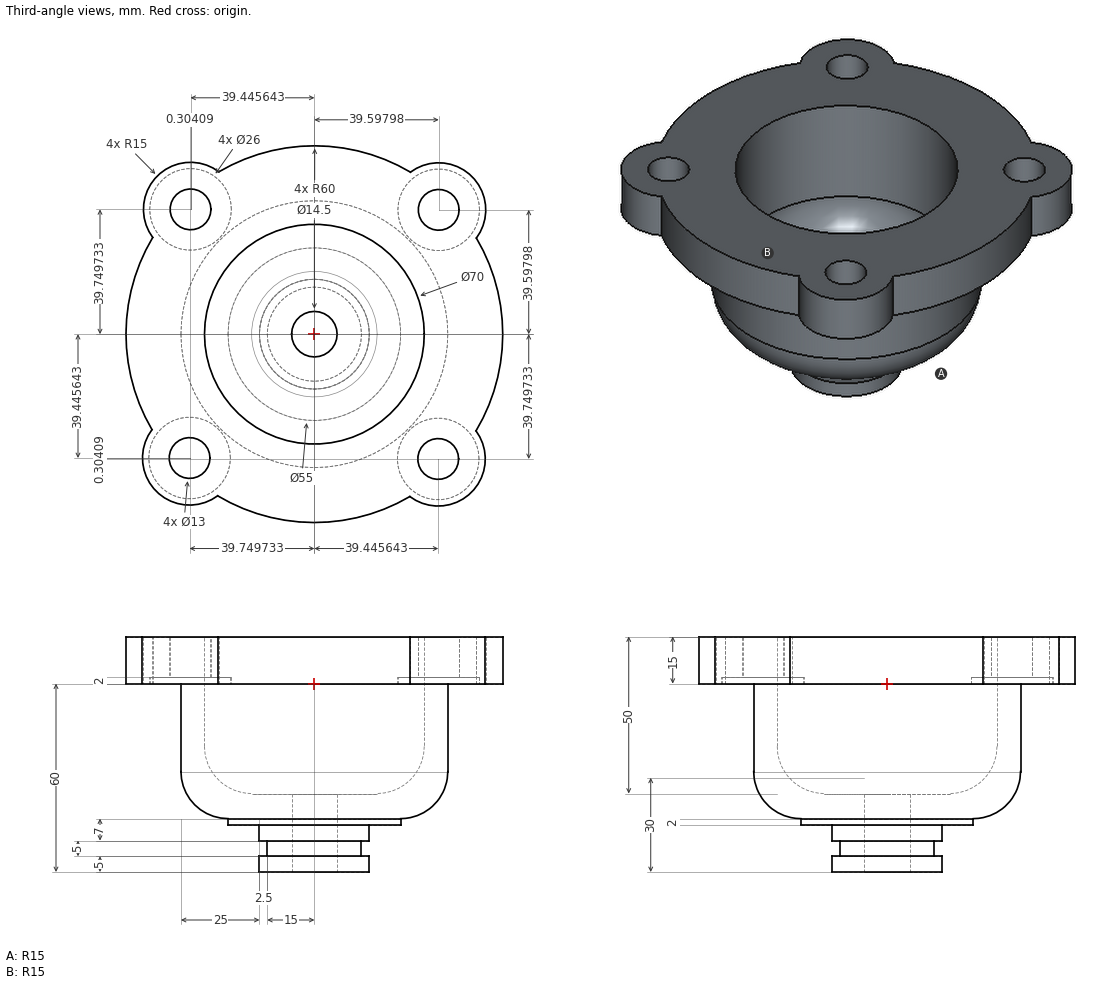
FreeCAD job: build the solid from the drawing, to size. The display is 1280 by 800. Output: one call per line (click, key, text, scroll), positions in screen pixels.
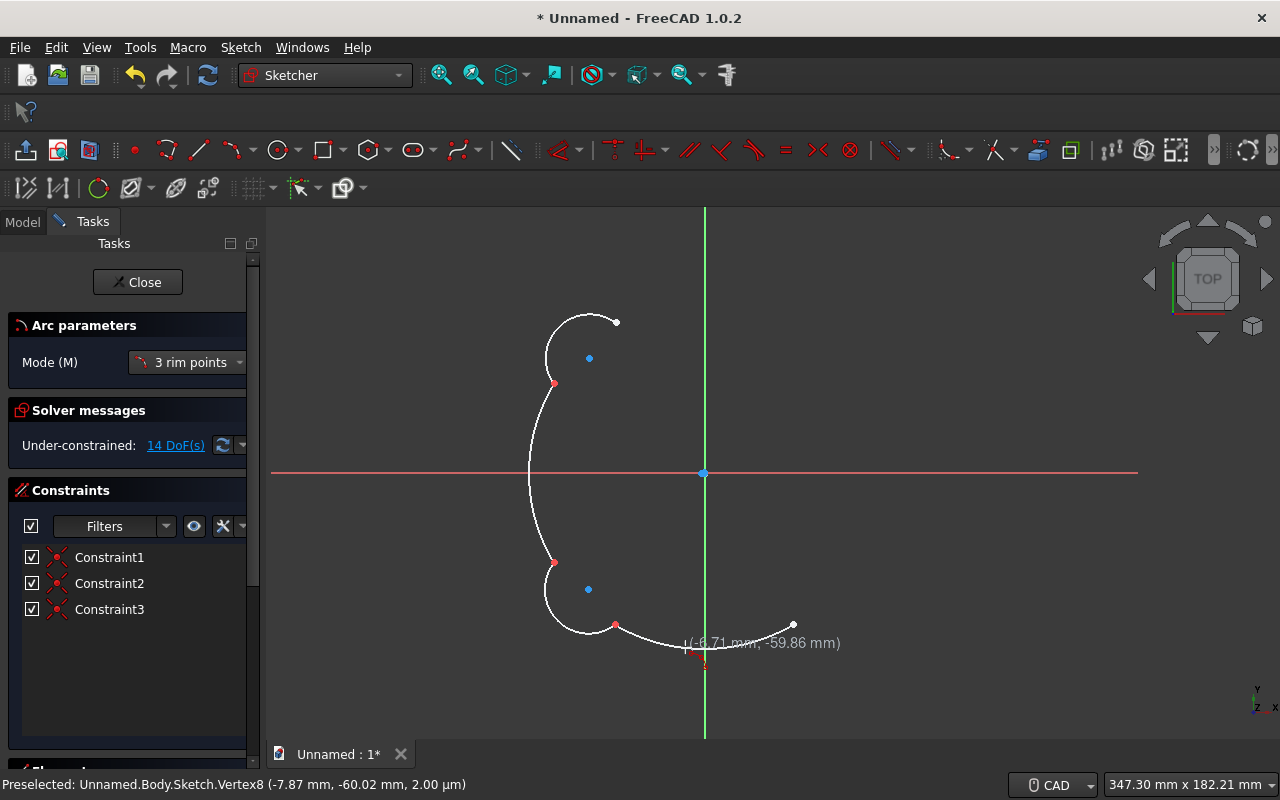
click(793, 625)
click(855, 563)
click(851, 620)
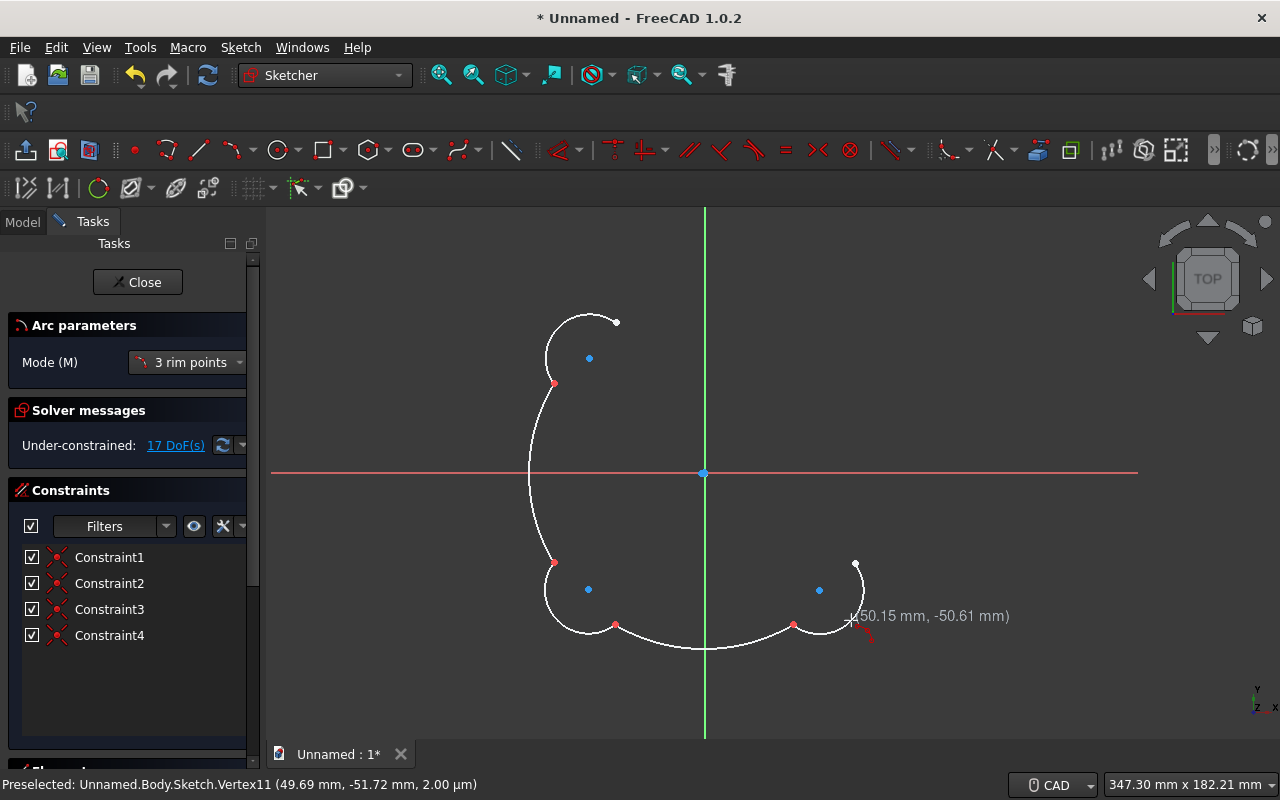
click(855, 564)
click(855, 384)
click(879, 492)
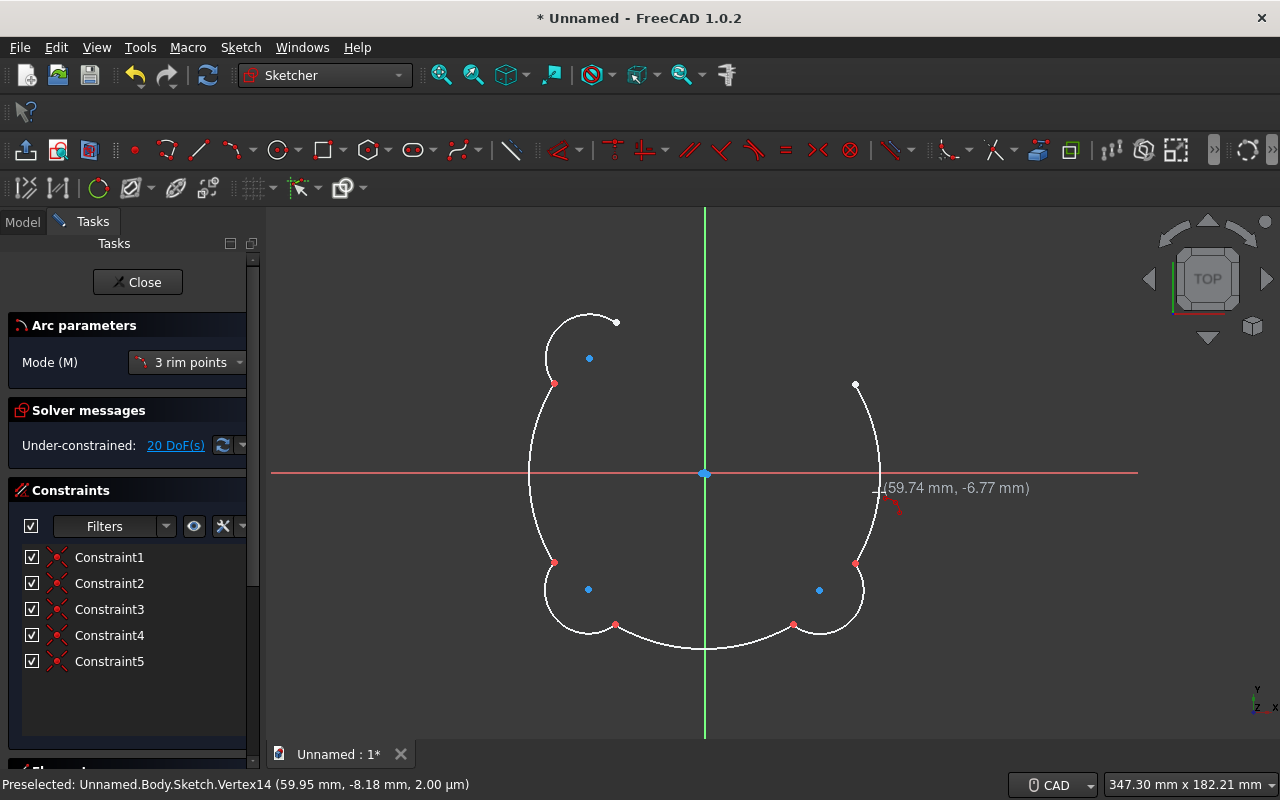
click(855, 385)
click(794, 323)
click(851, 327)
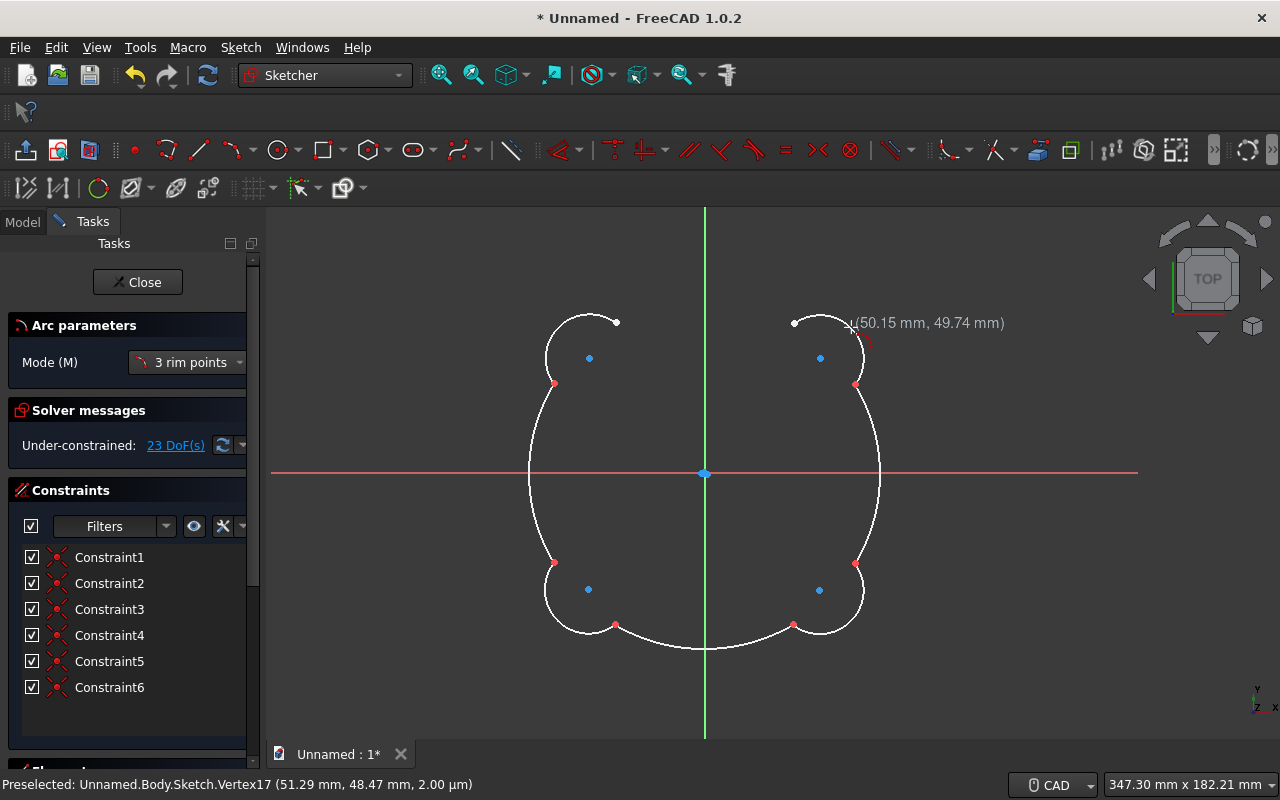
click(794, 324)
click(616, 323)
click(724, 299)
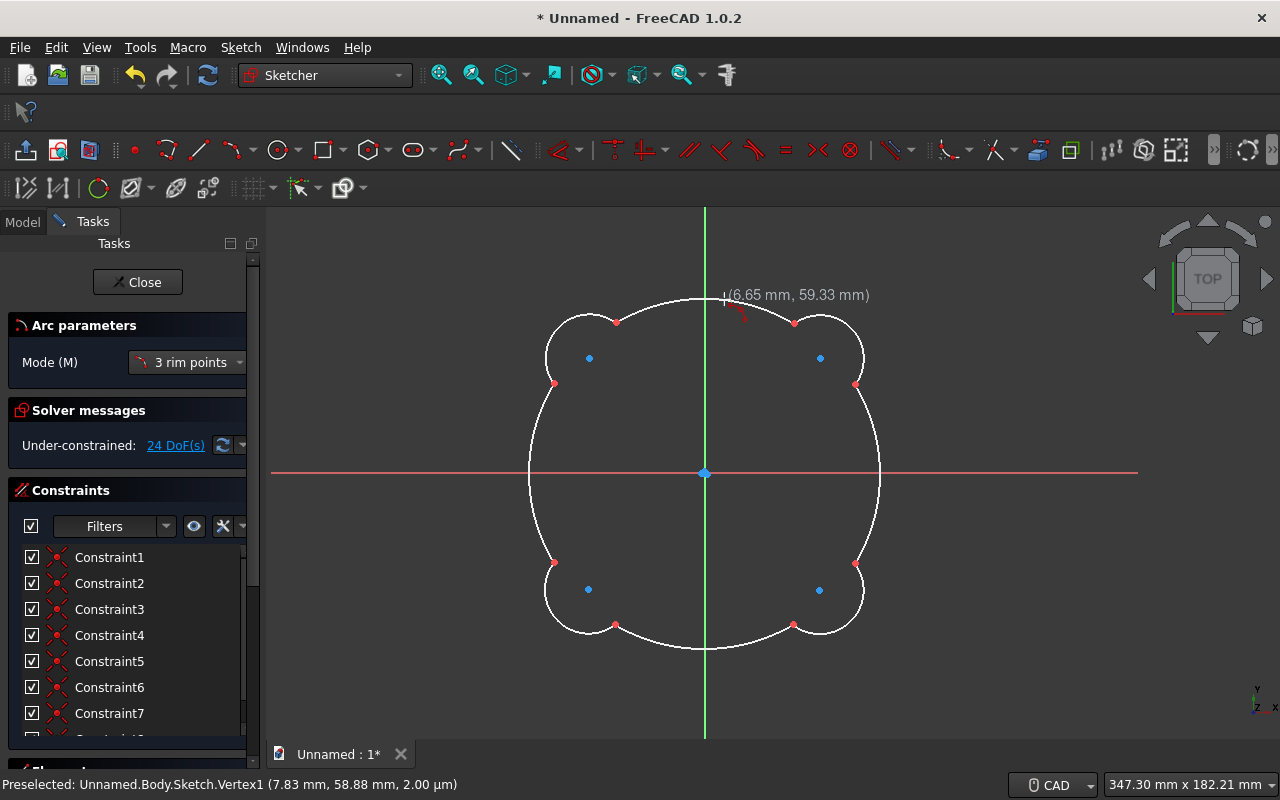
click(278, 150)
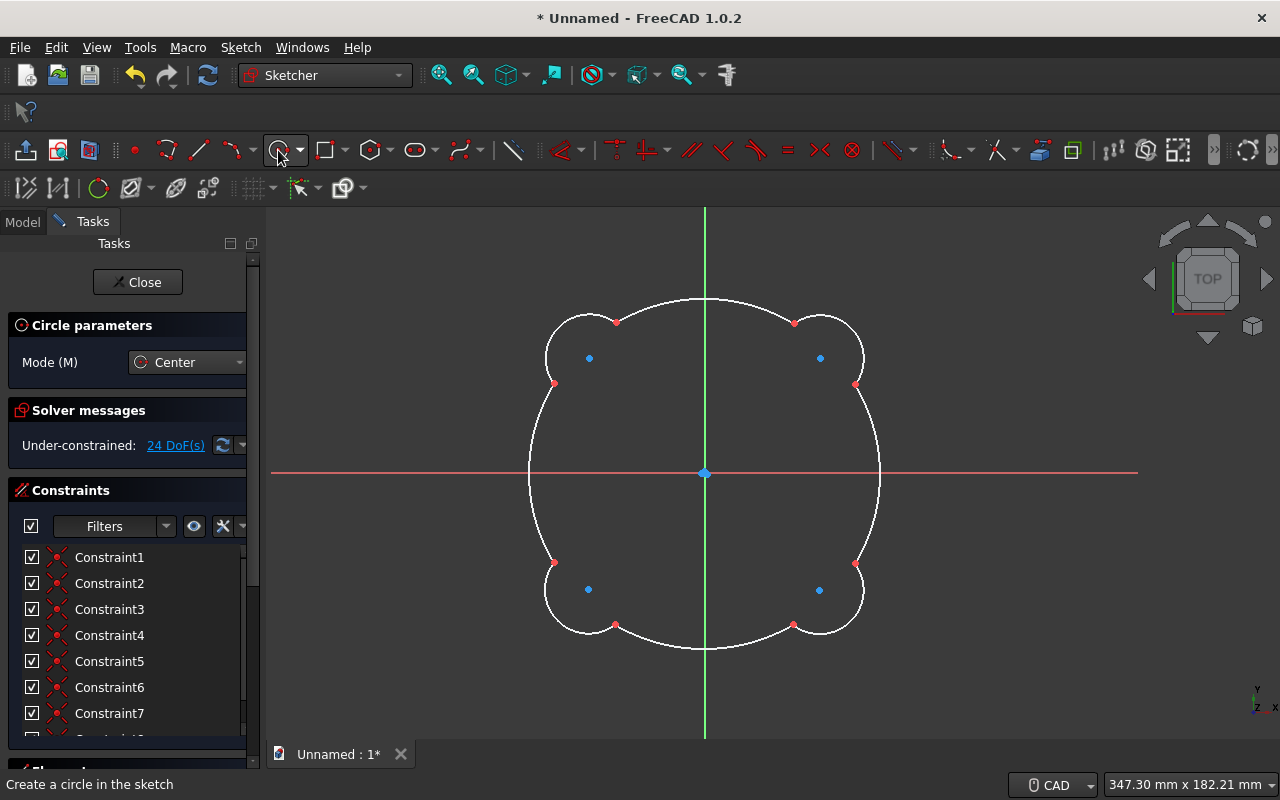
click(589, 588)
move(602, 575)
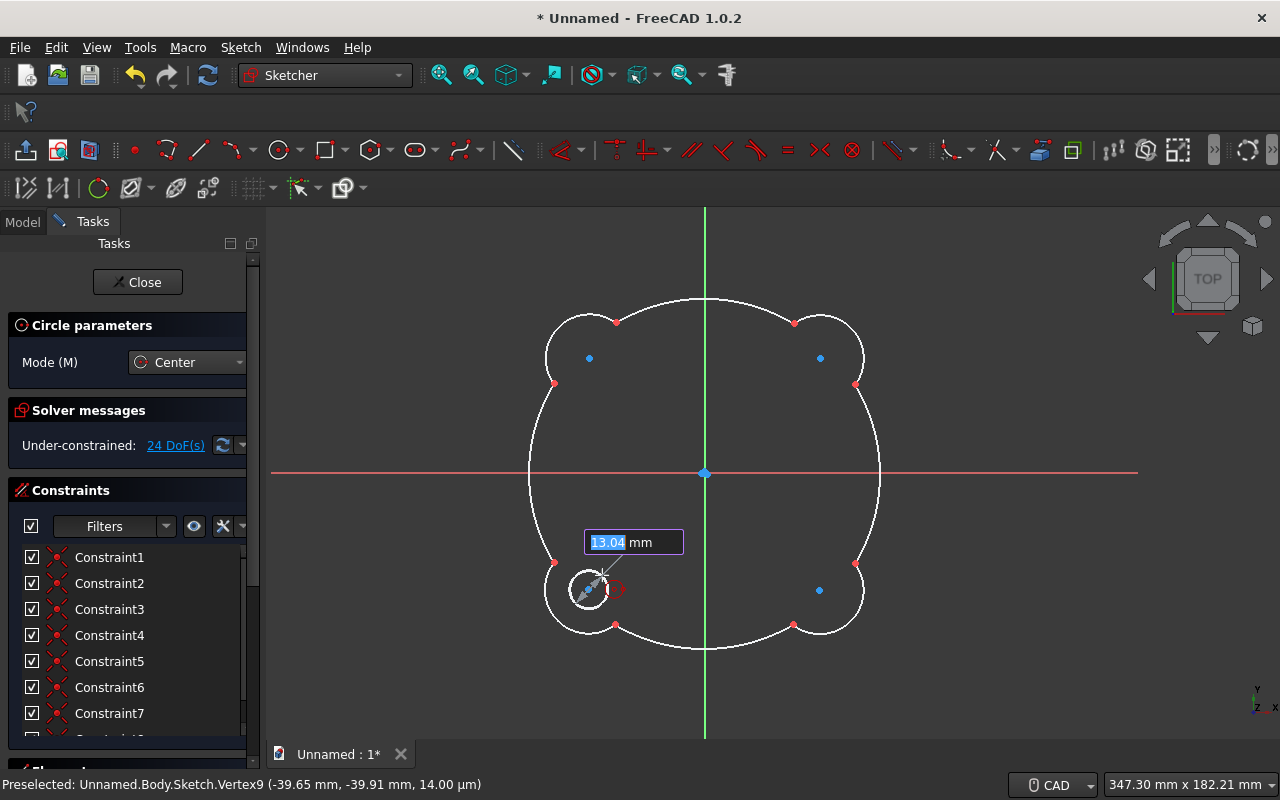
text(13)
key(Return)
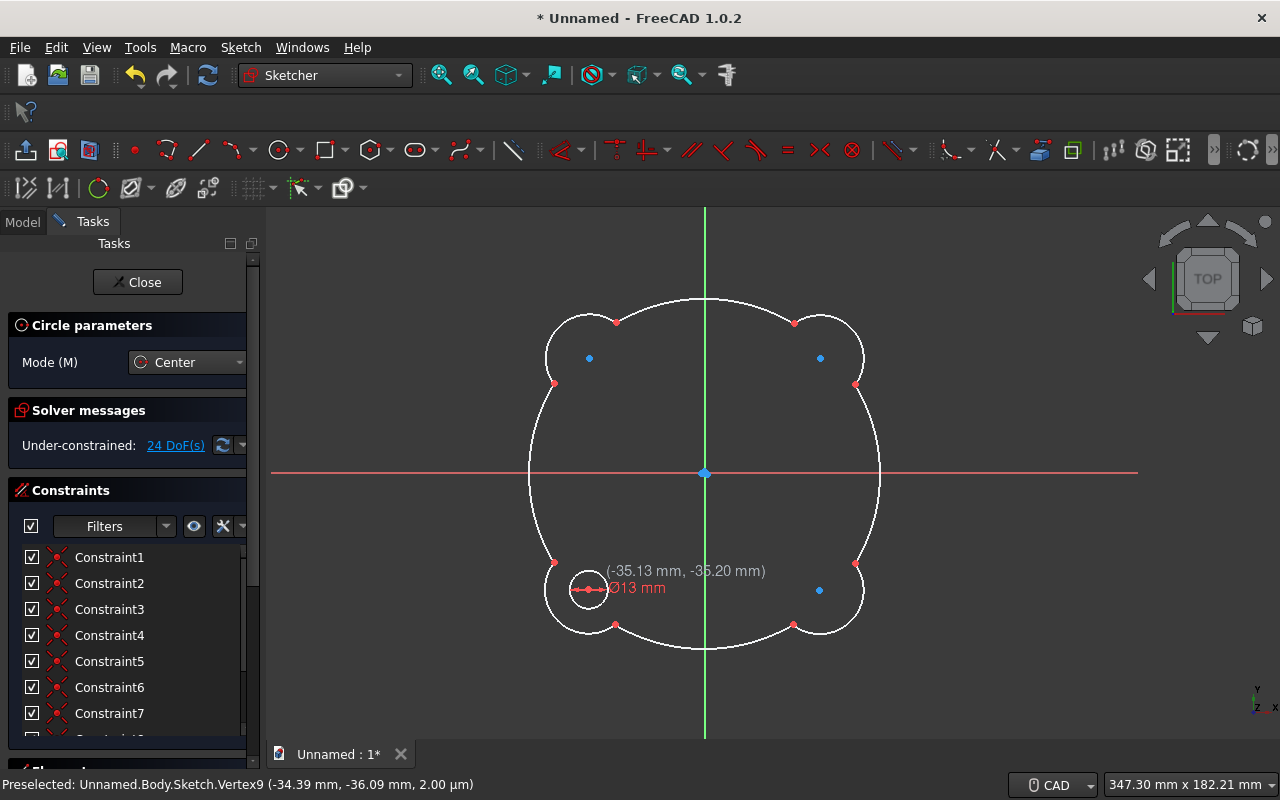
click(820, 589)
move(833, 576)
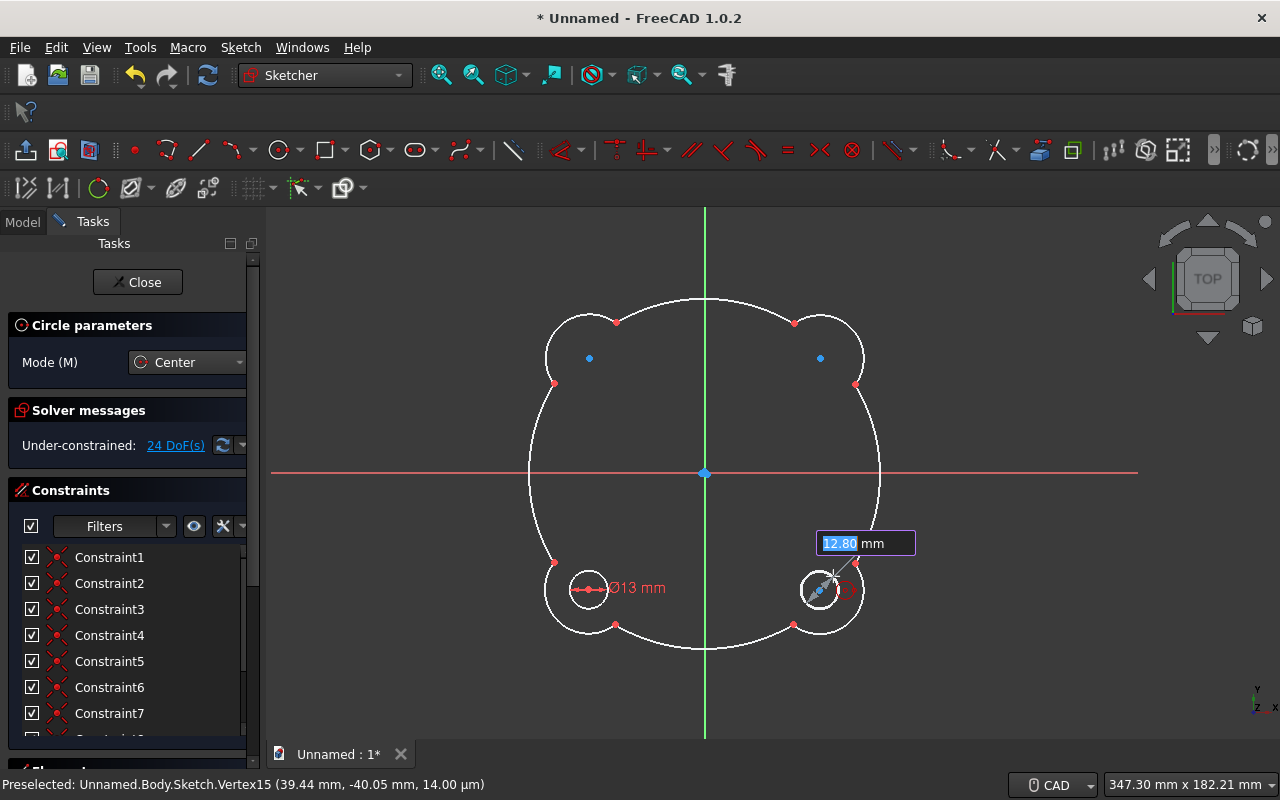
text(13)
key(Return)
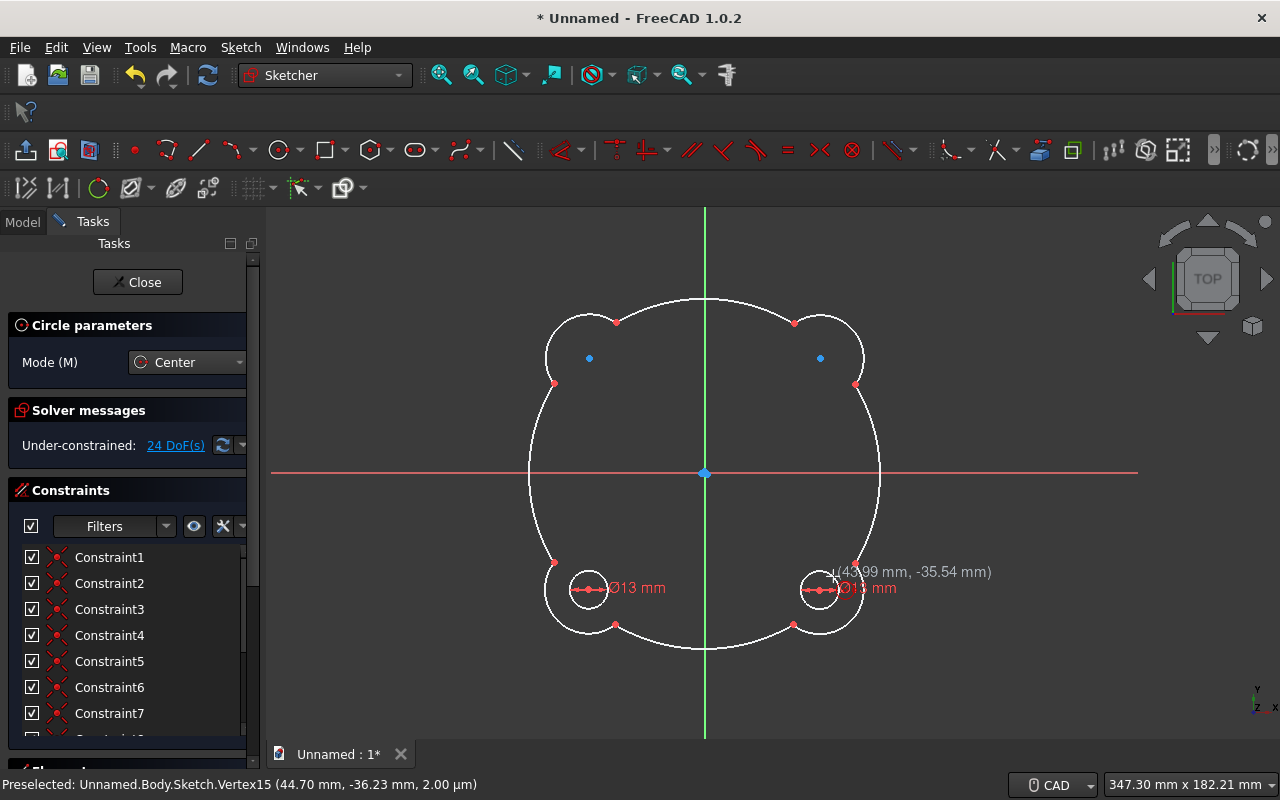
click(589, 357)
move(603, 344)